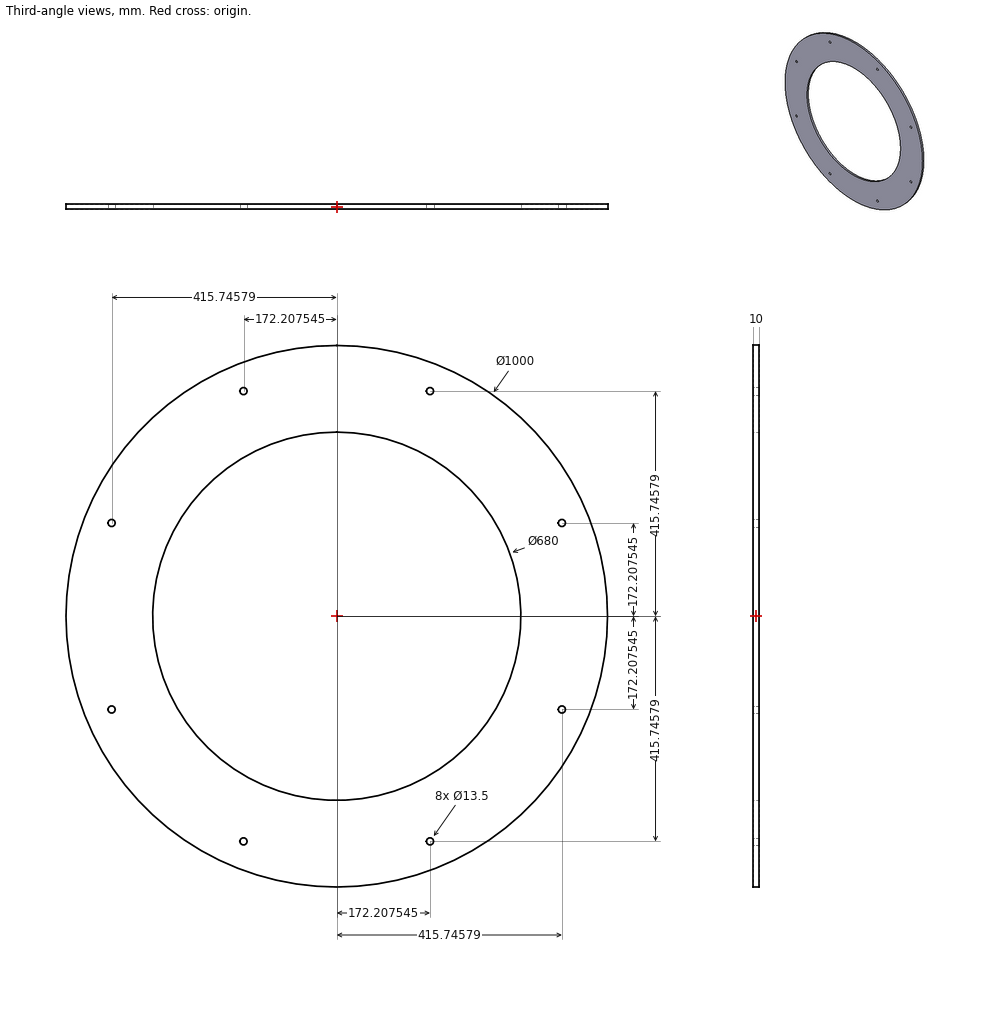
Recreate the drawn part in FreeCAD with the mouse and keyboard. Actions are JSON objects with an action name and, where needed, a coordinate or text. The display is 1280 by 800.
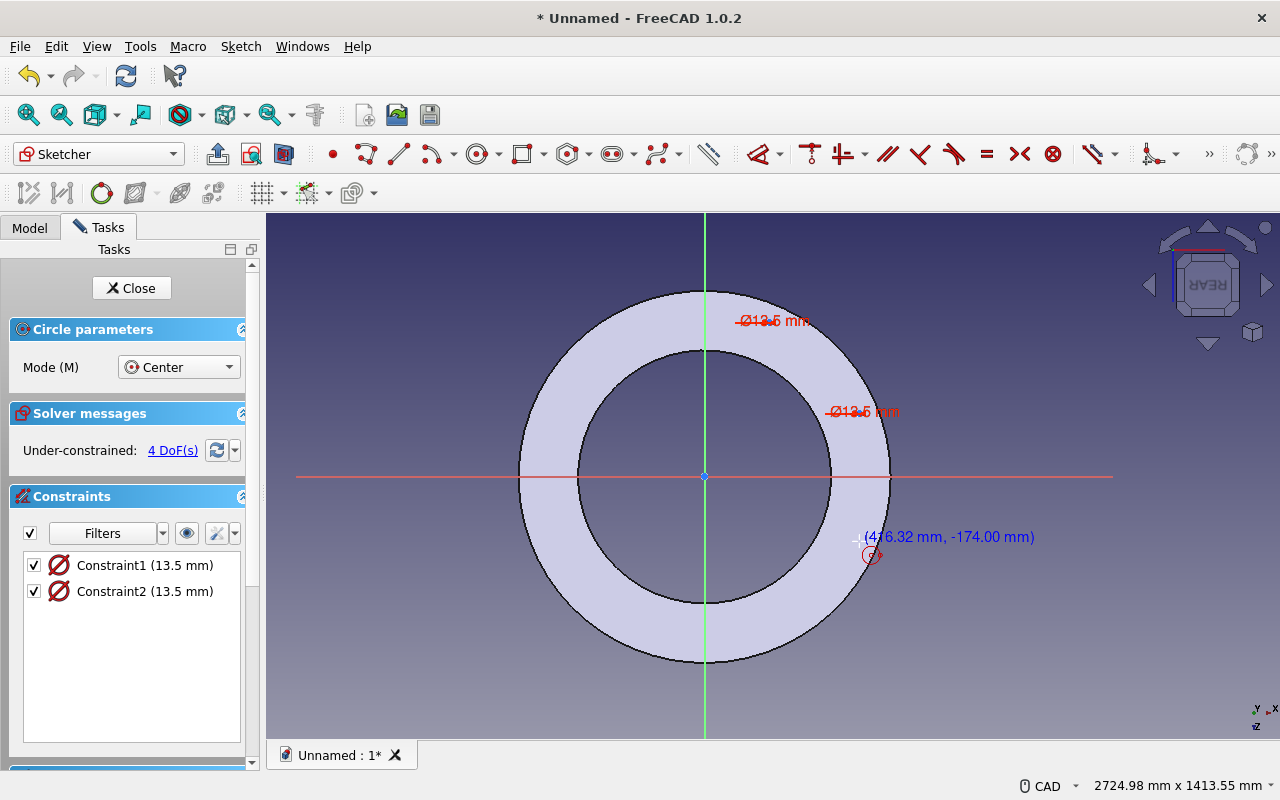
{"action": "left_click", "coordinate": [859, 541]}
{"action": "mouse_move", "coordinate": [861, 539]}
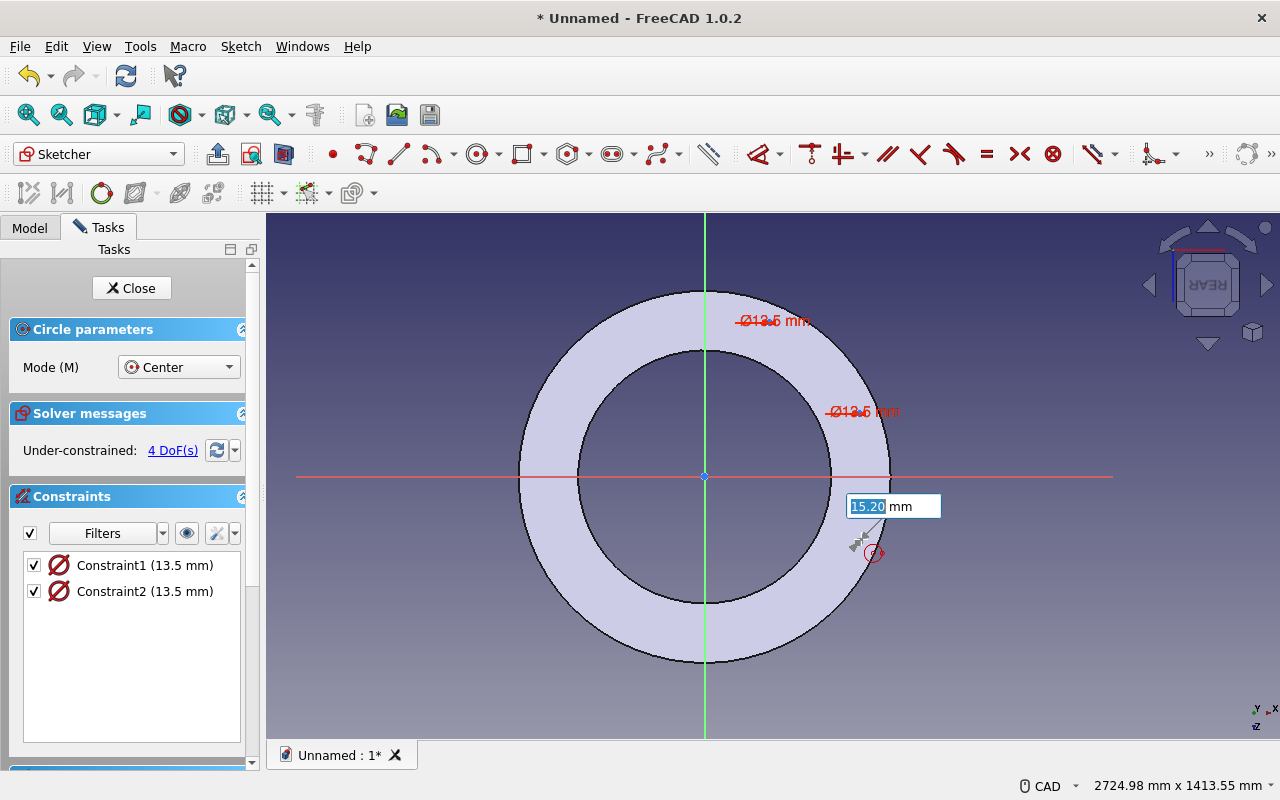
{"action": "type", "text": "13.5"}
{"action": "key", "text": "Return"}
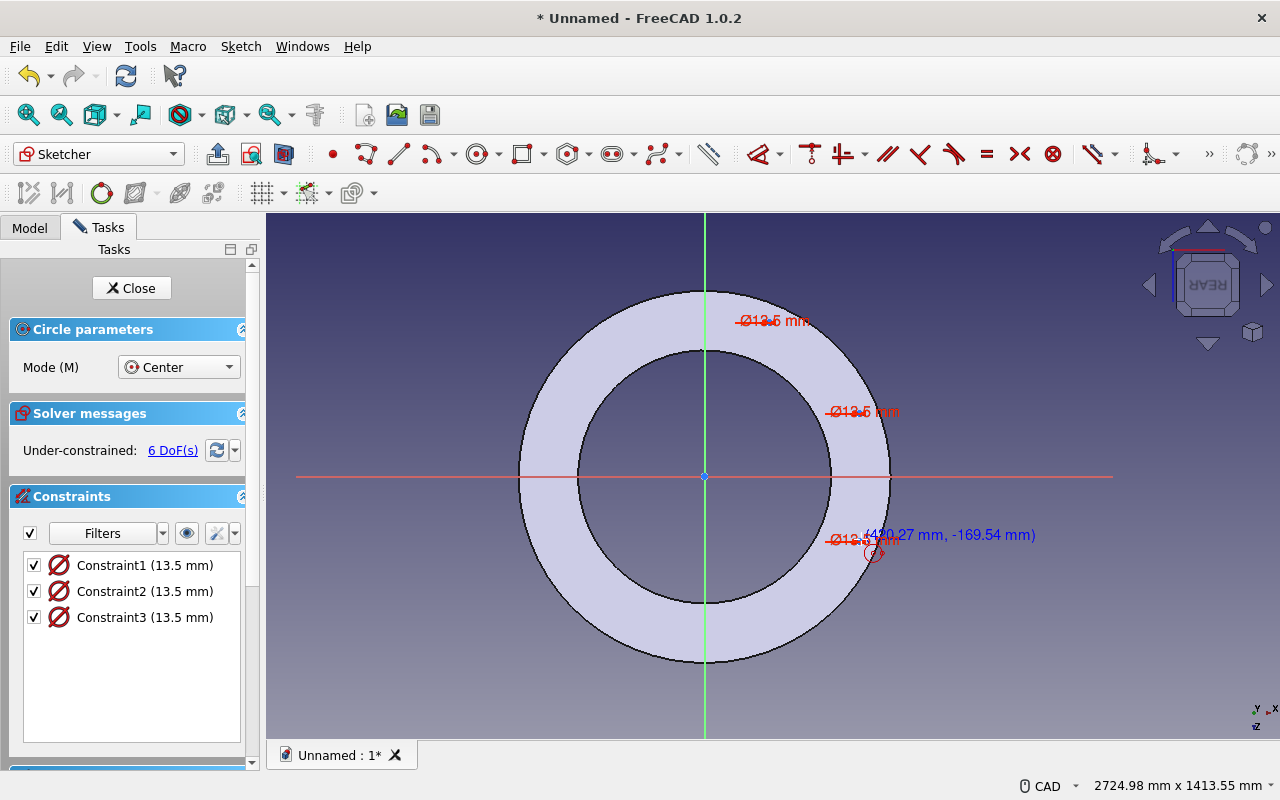
{"action": "scroll", "coordinate": [769, 632], "scroll_direction": "up", "scroll_amount": 12}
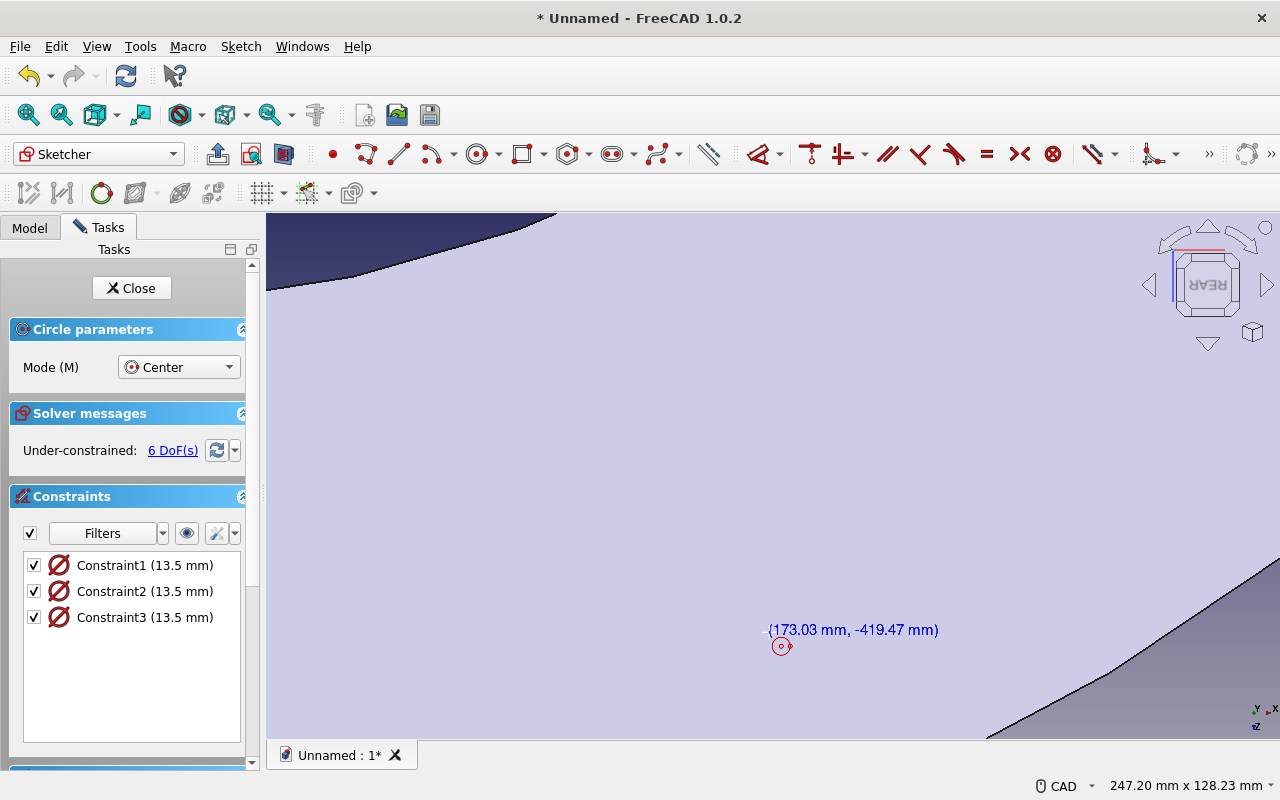
{"action": "scroll", "coordinate": [769, 632], "scroll_direction": "down", "scroll_amount": 12}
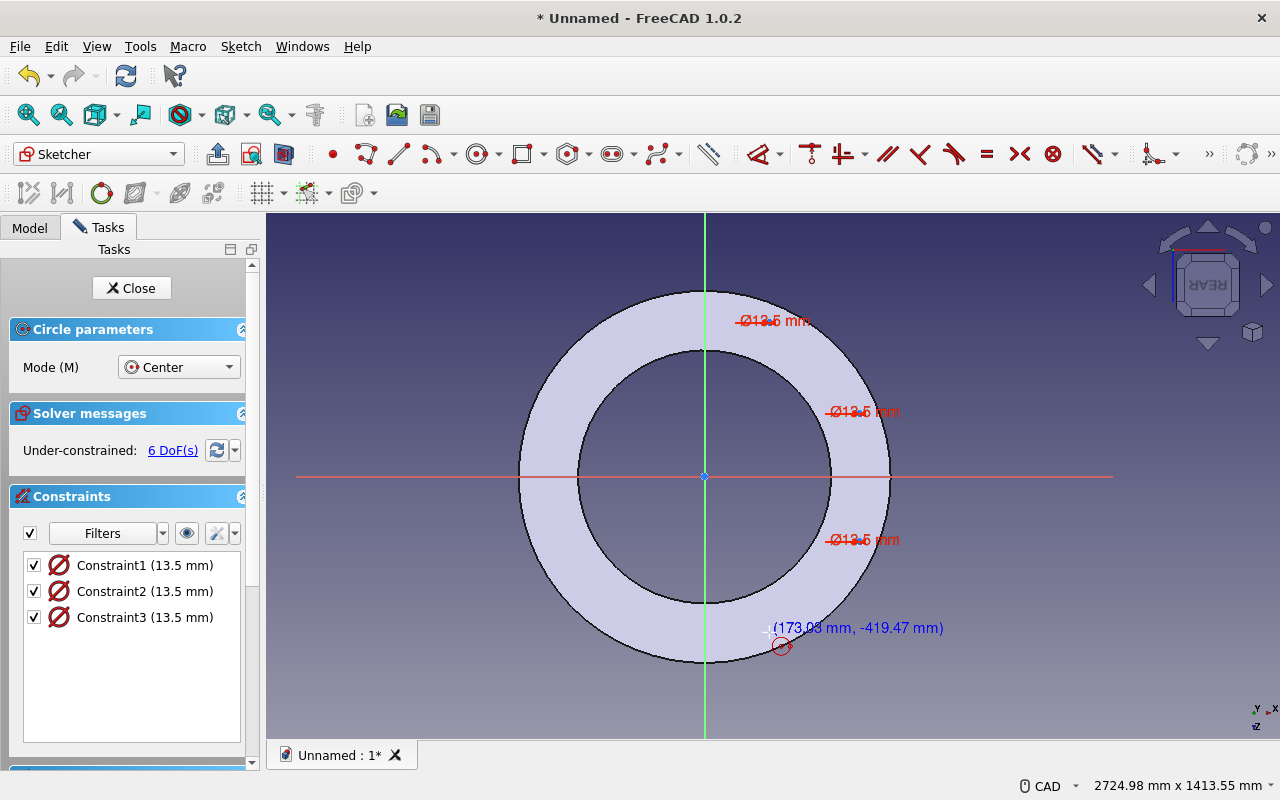
{"action": "left_click", "coordinate": [769, 632]}
{"action": "mouse_move", "coordinate": [770, 630]}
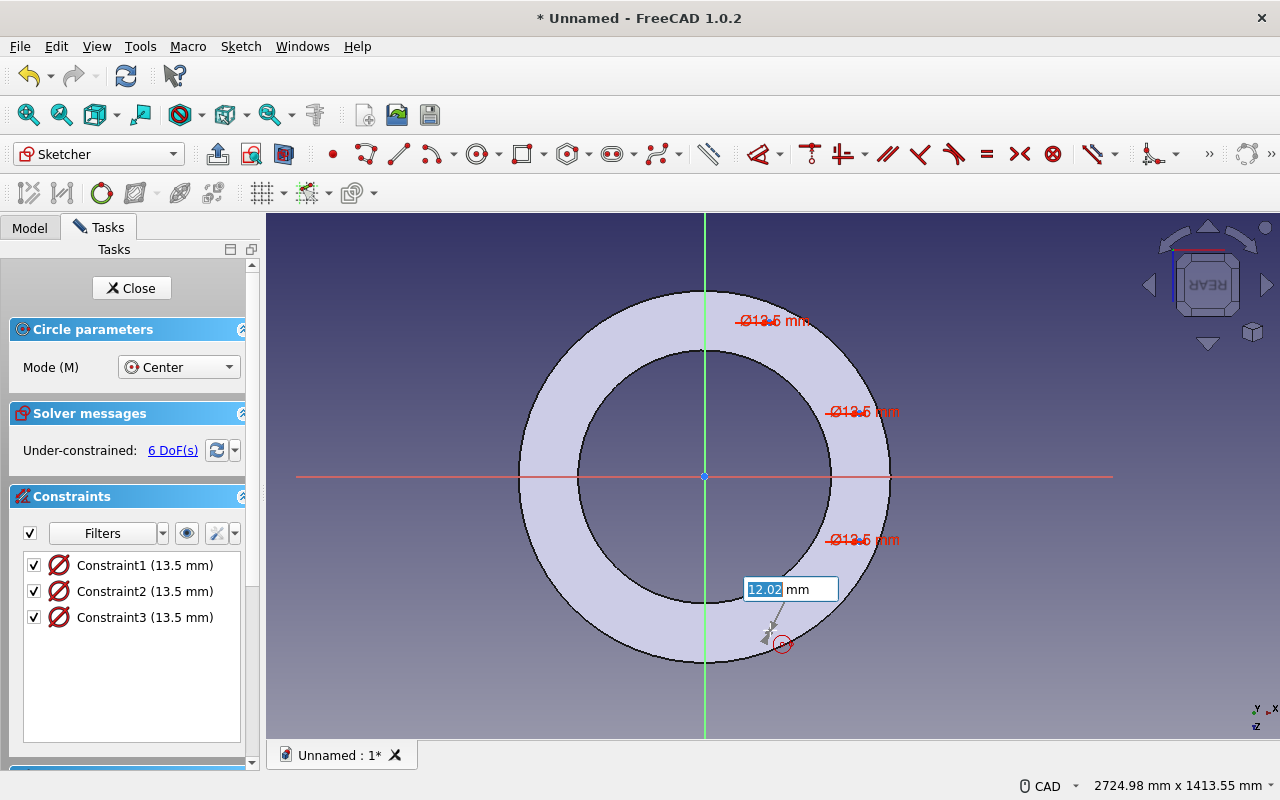
{"action": "type", "text": "13.5"}
{"action": "key", "text": "Return"}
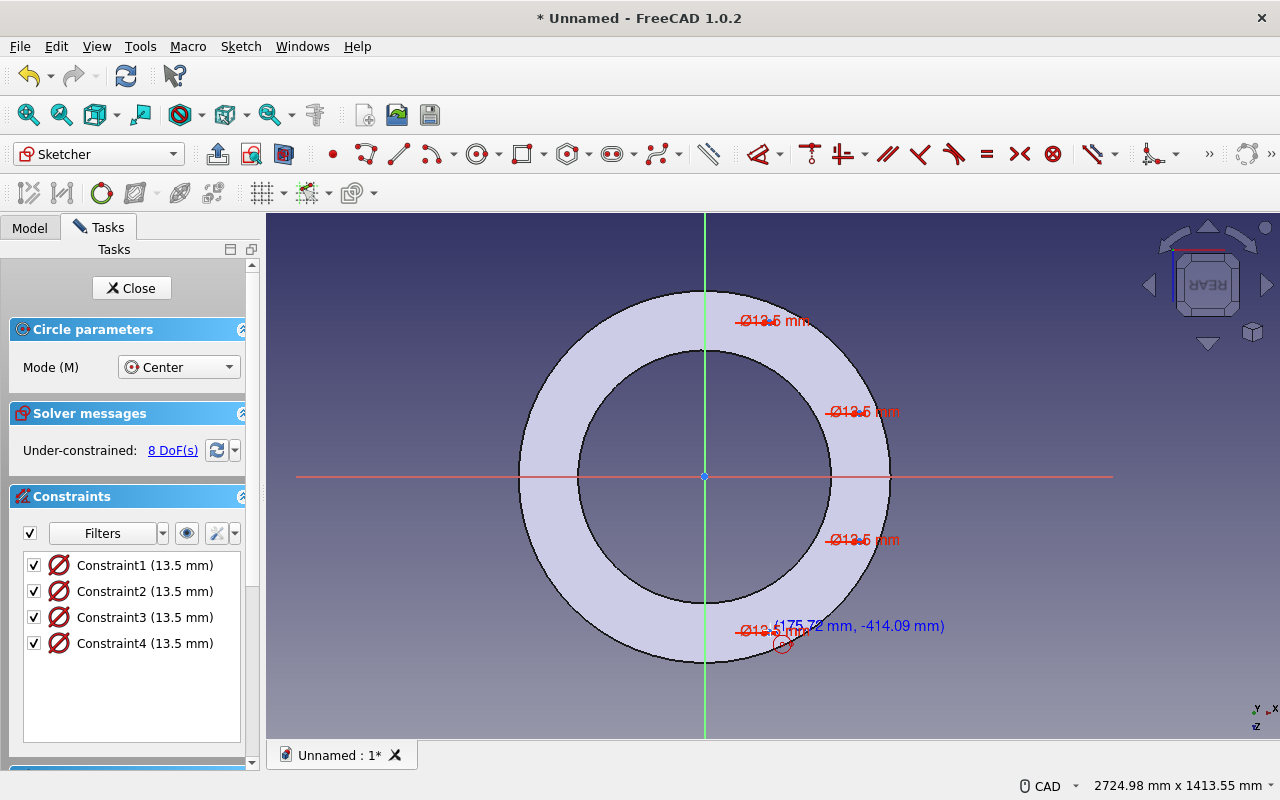
{"action": "scroll", "coordinate": [641, 632], "scroll_direction": "up", "scroll_amount": 12}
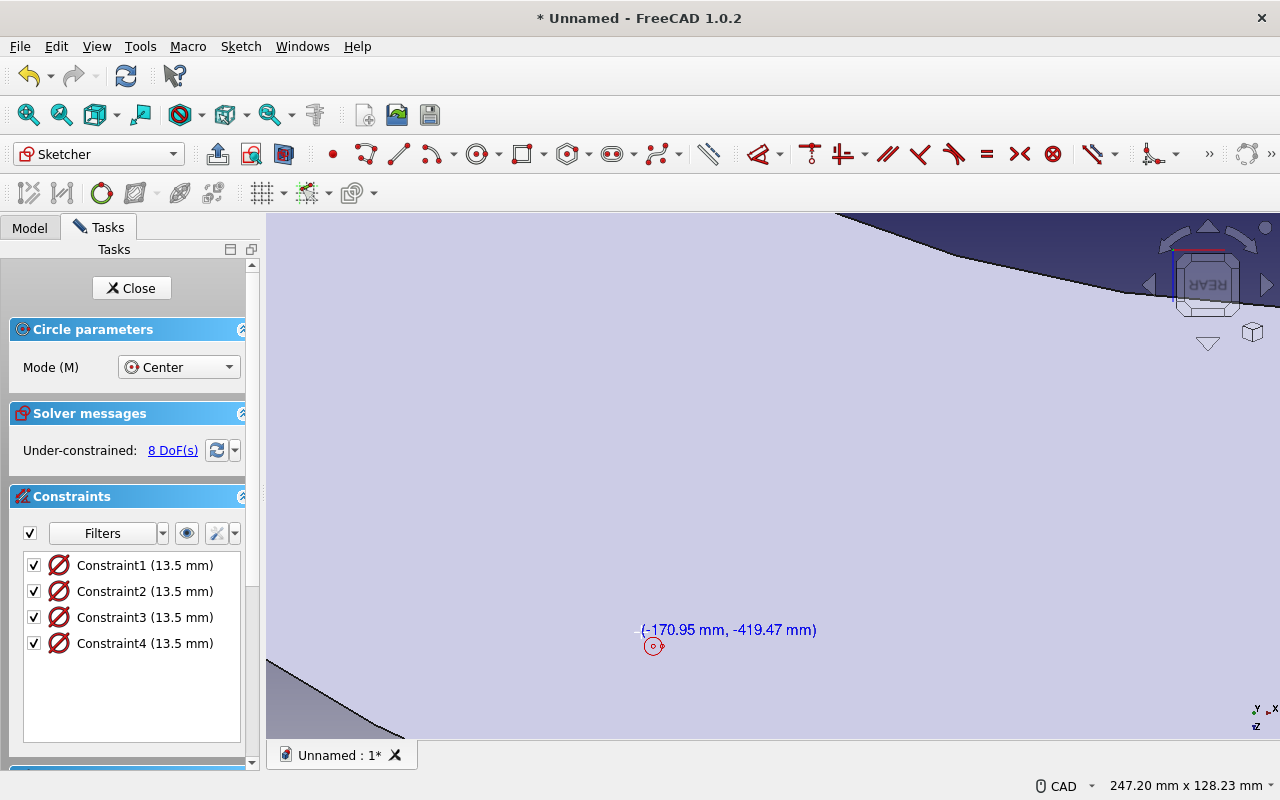
{"action": "scroll", "coordinate": [641, 632], "scroll_direction": "down", "scroll_amount": 12}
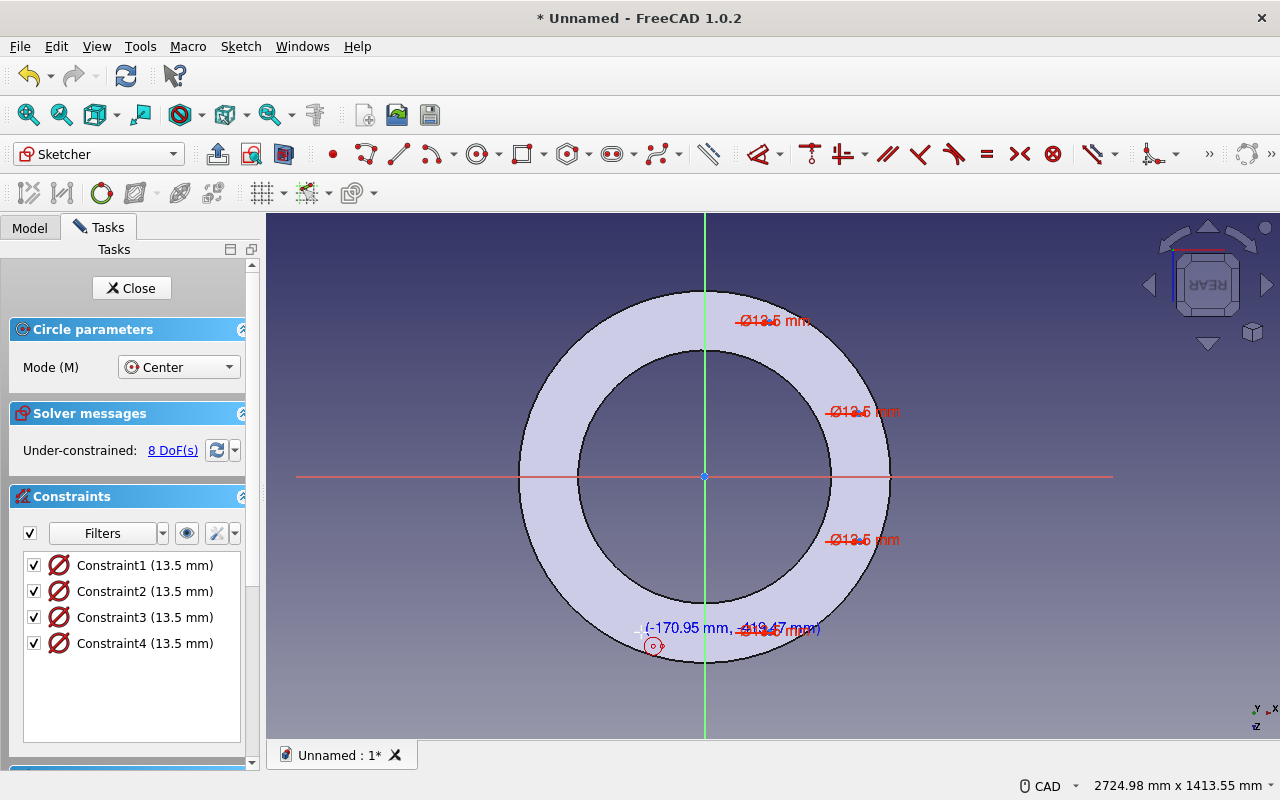
{"action": "left_click", "coordinate": [641, 632]}
{"action": "mouse_move", "coordinate": [642, 630]}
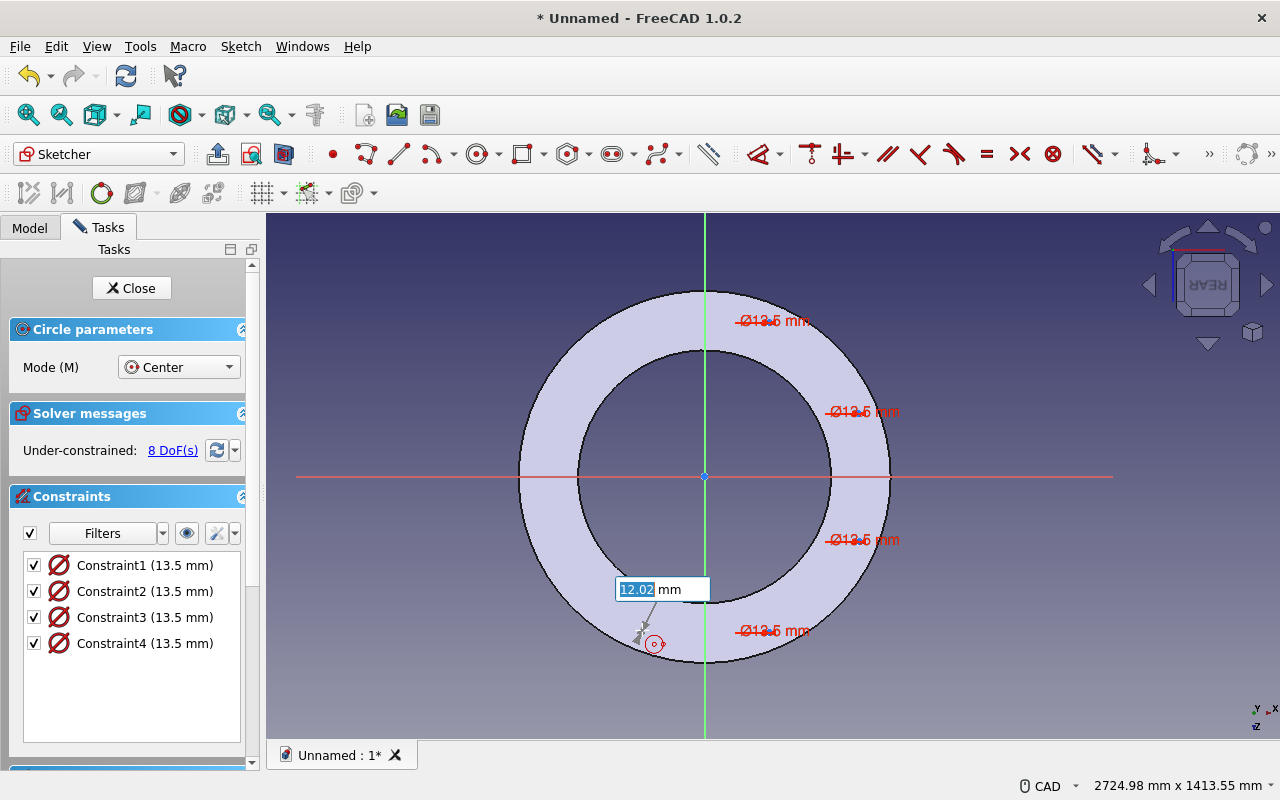
{"action": "type", "text": "13.5"}
{"action": "key", "text": "Return"}